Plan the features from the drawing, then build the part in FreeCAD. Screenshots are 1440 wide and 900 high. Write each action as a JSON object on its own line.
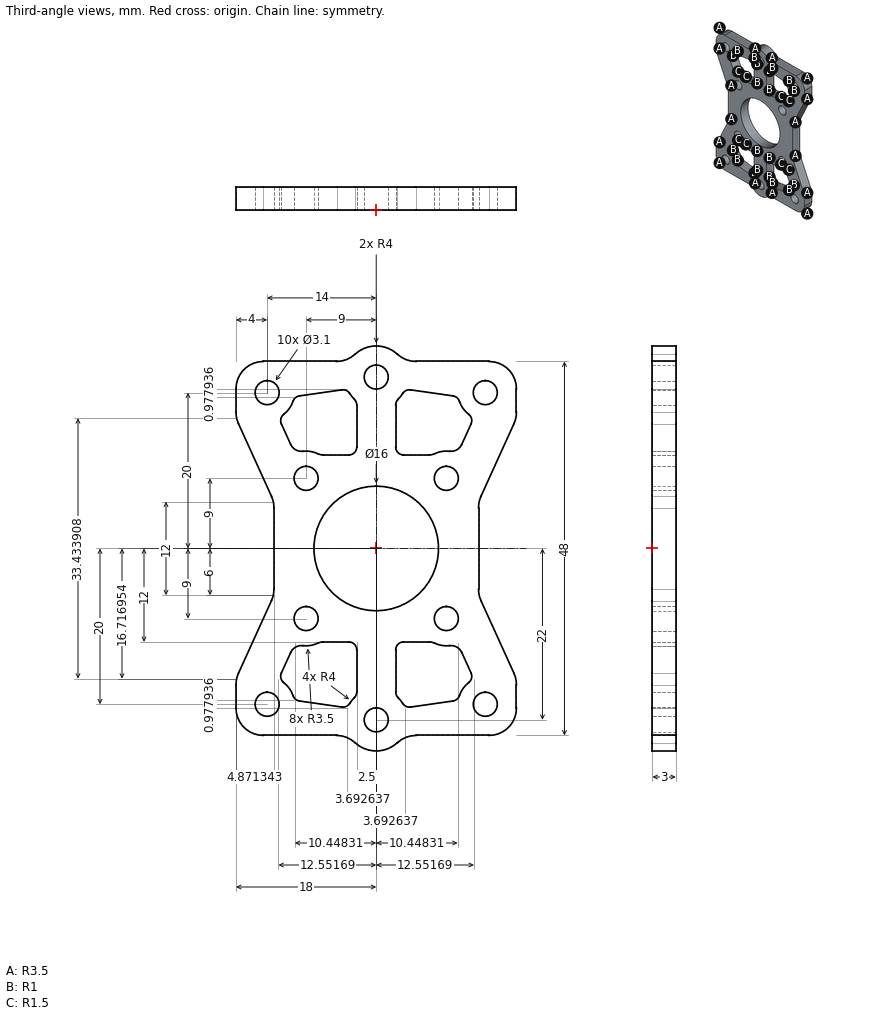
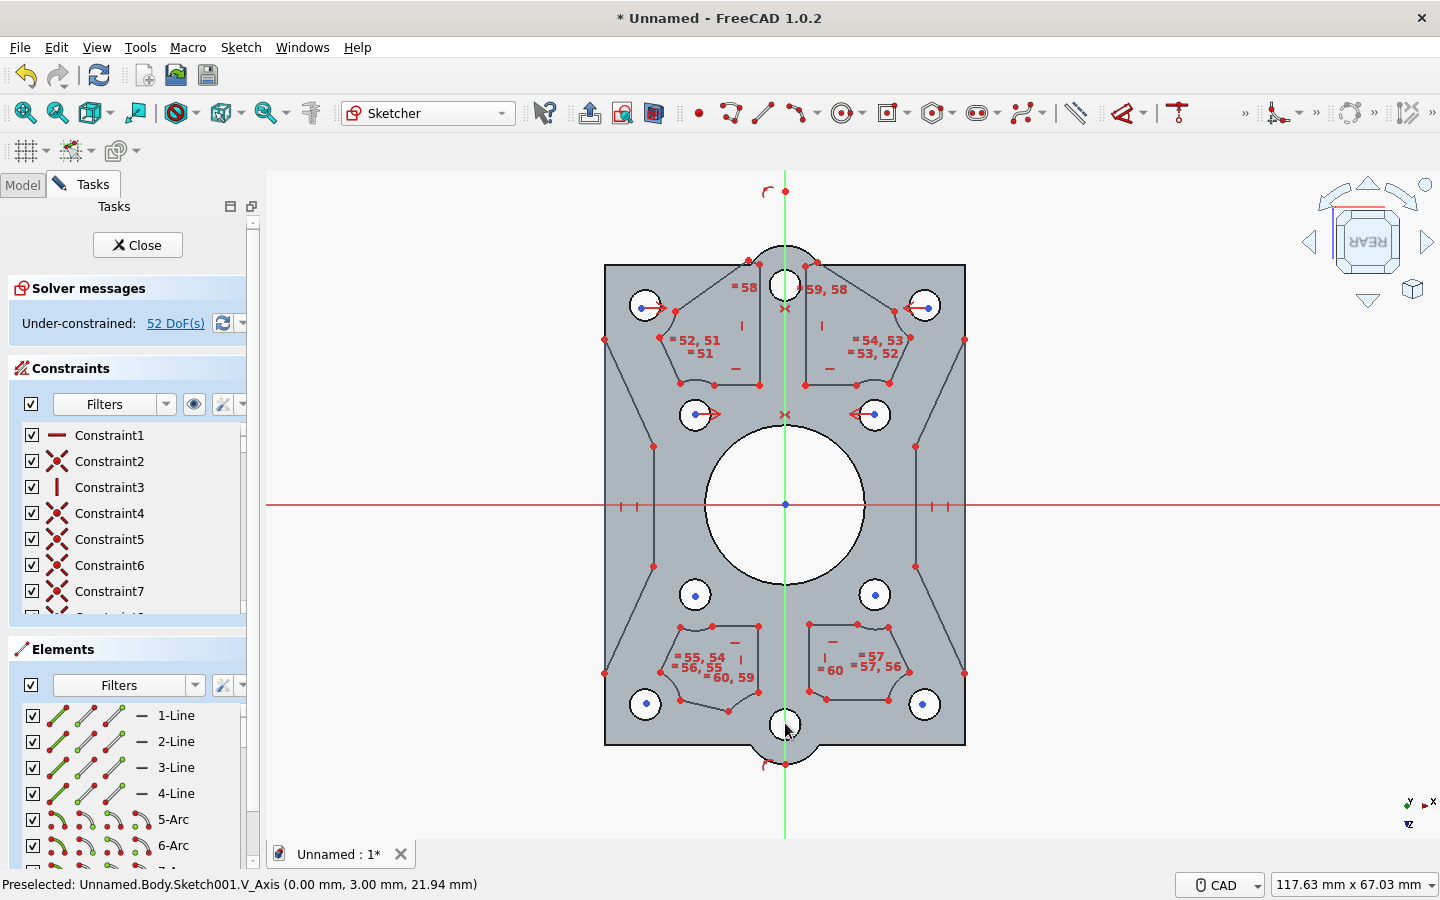
{"action": "left_click", "coordinate": [695, 414]}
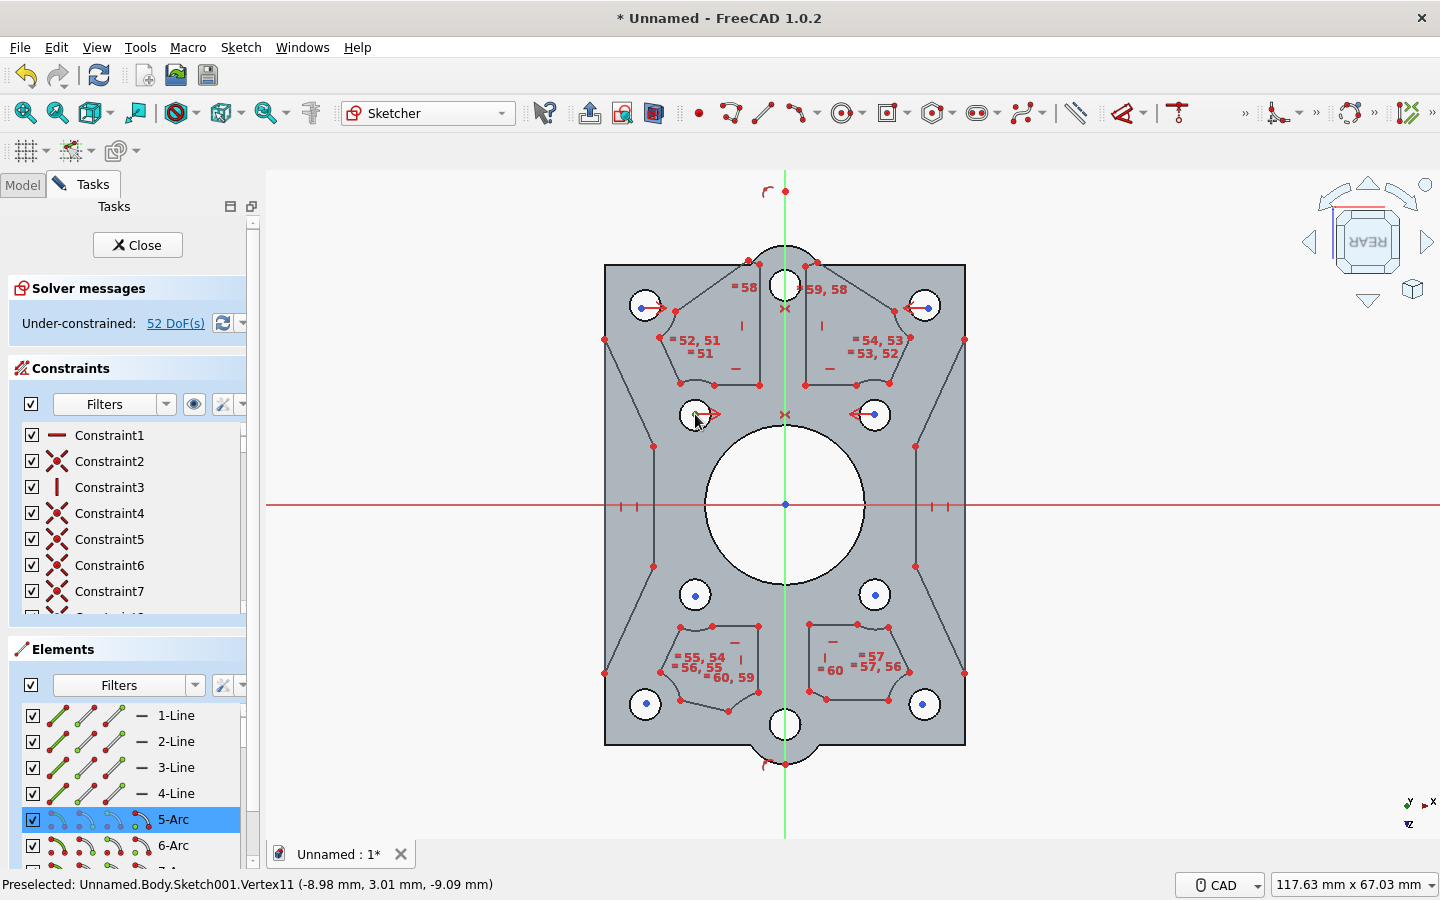
{"action": "left_click", "coordinate": [696, 596]}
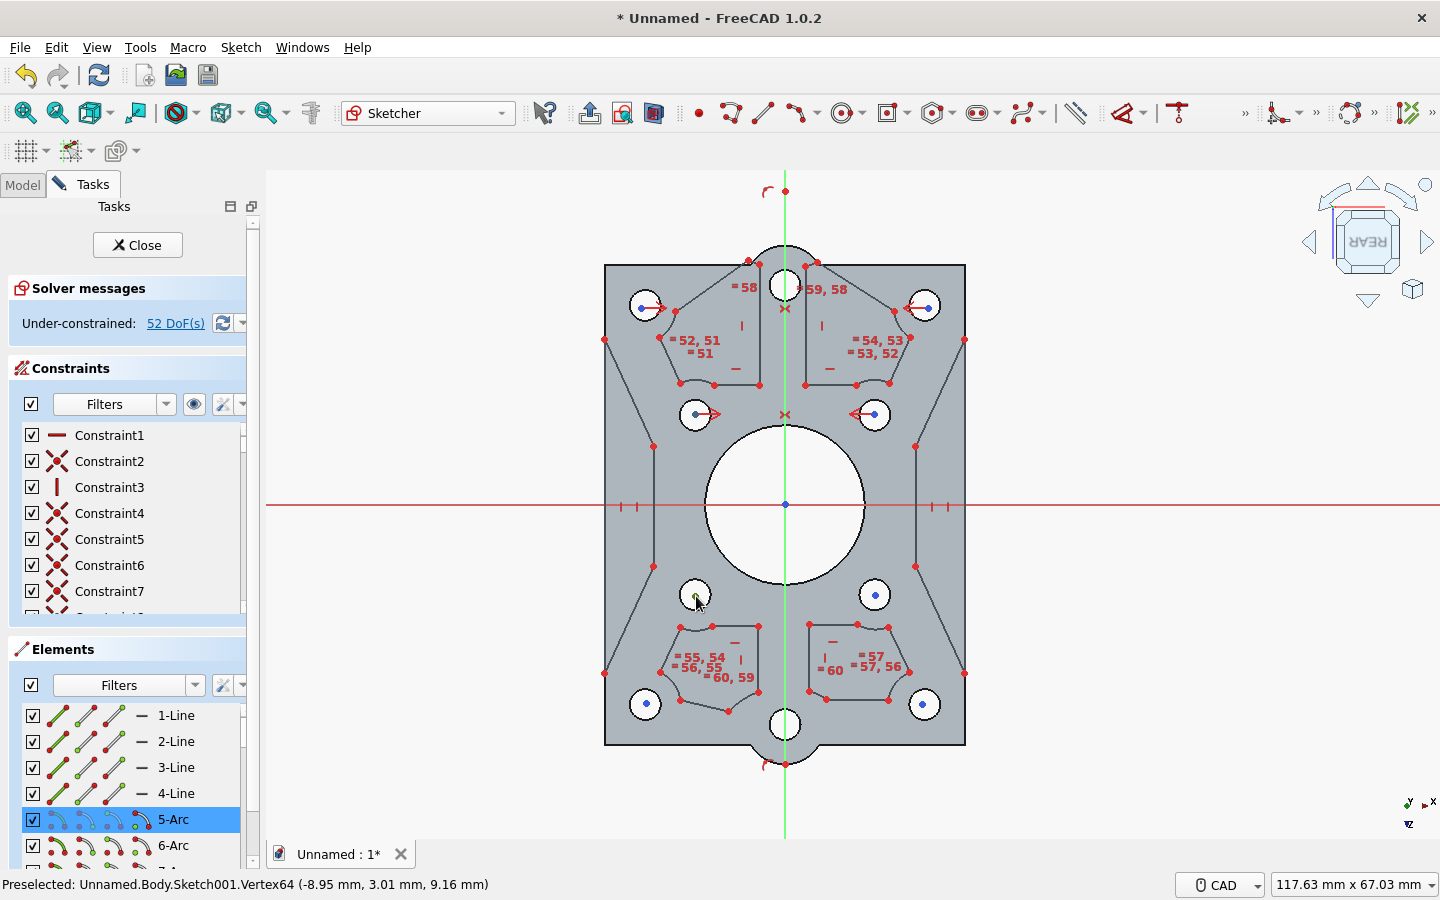
{"action": "left_click", "coordinate": [364, 505]}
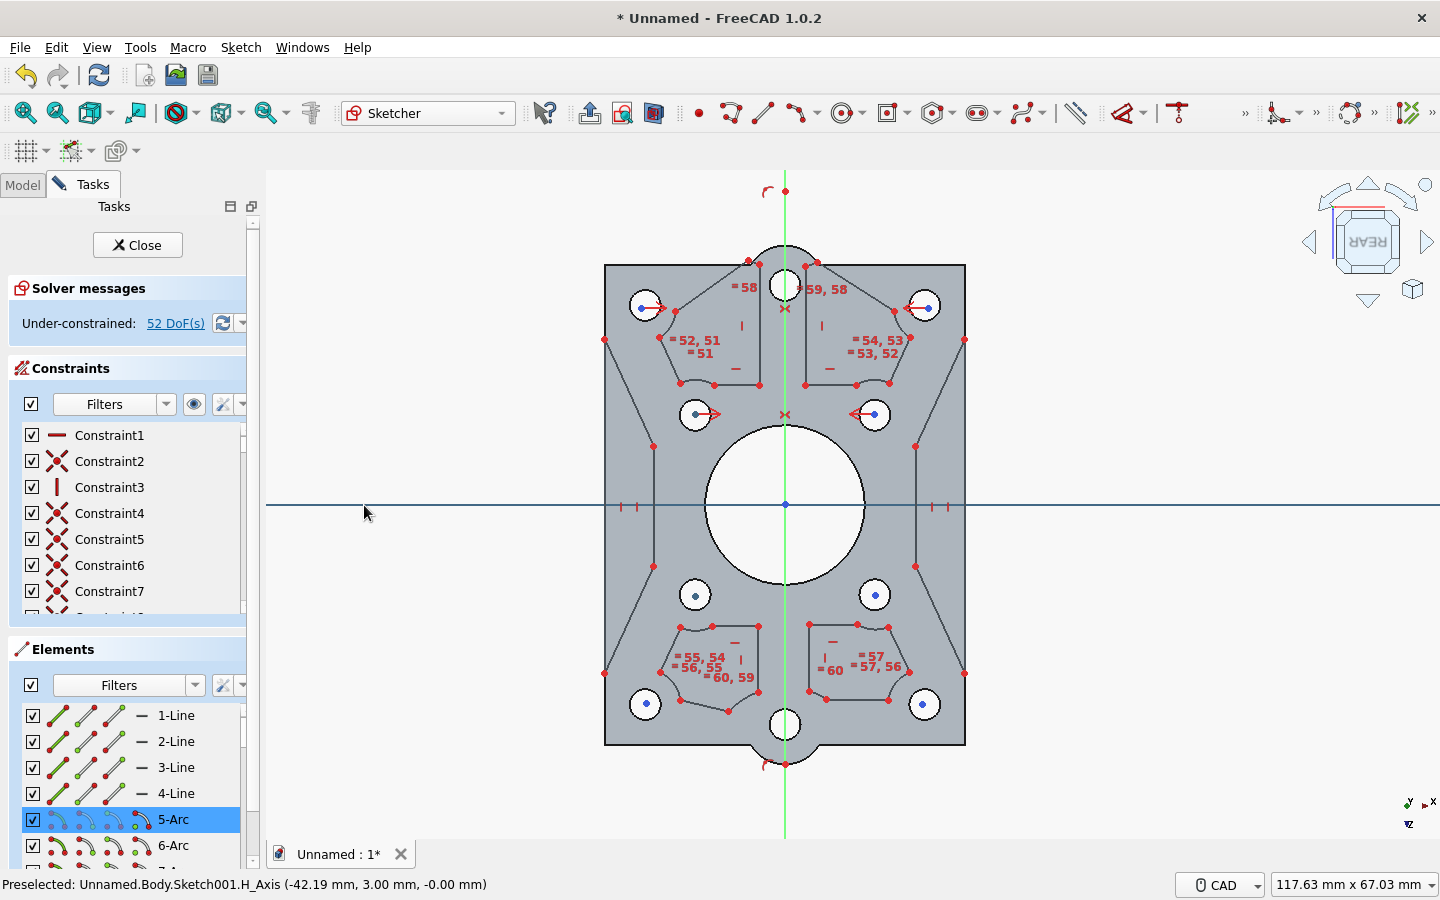
{"action": "key", "text": "s"}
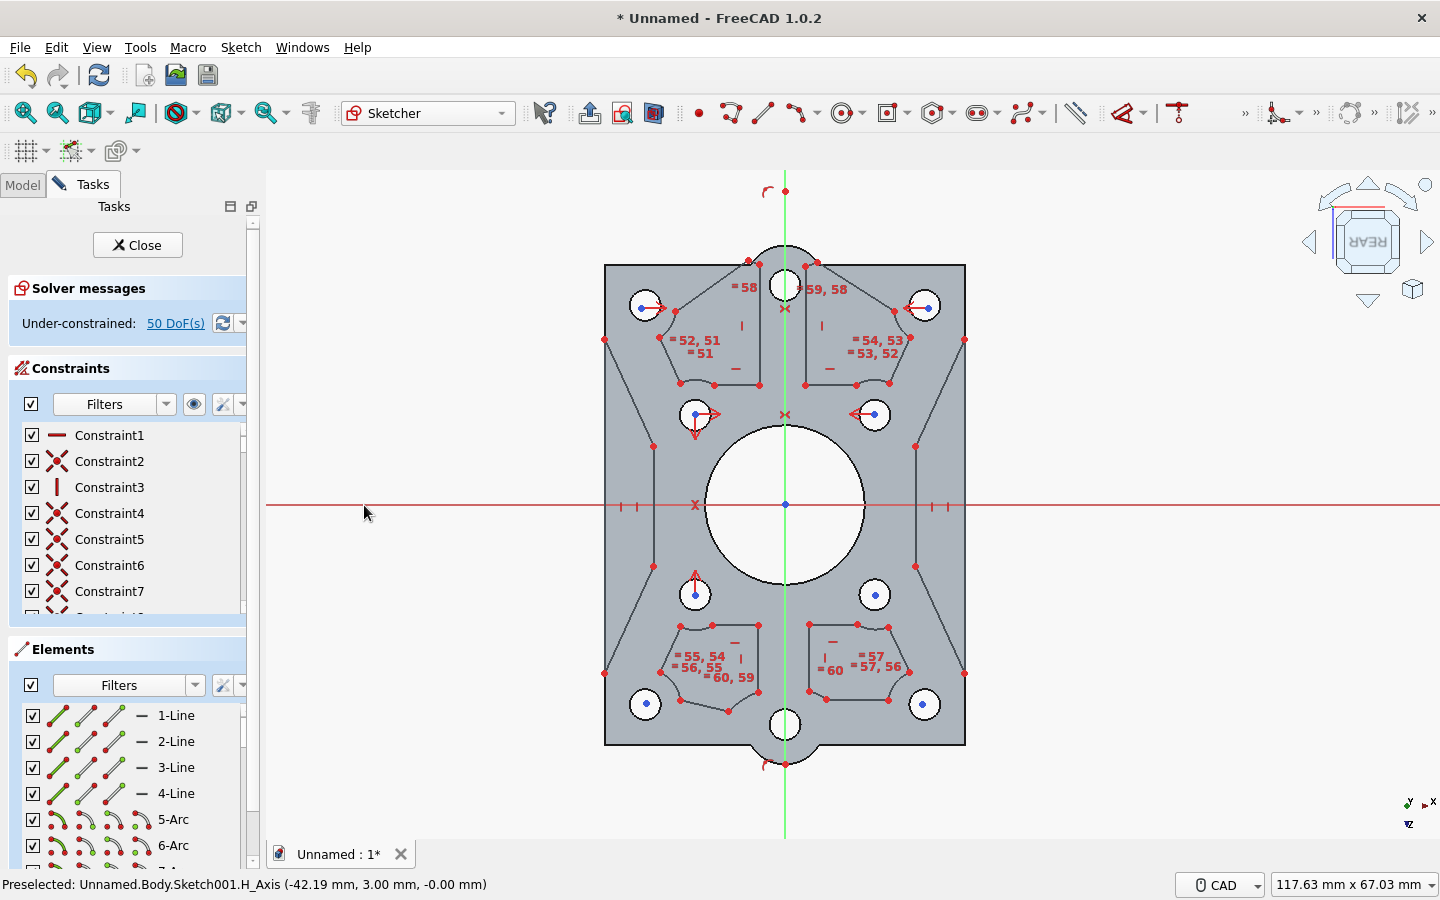
{"action": "left_click", "coordinate": [642, 308]}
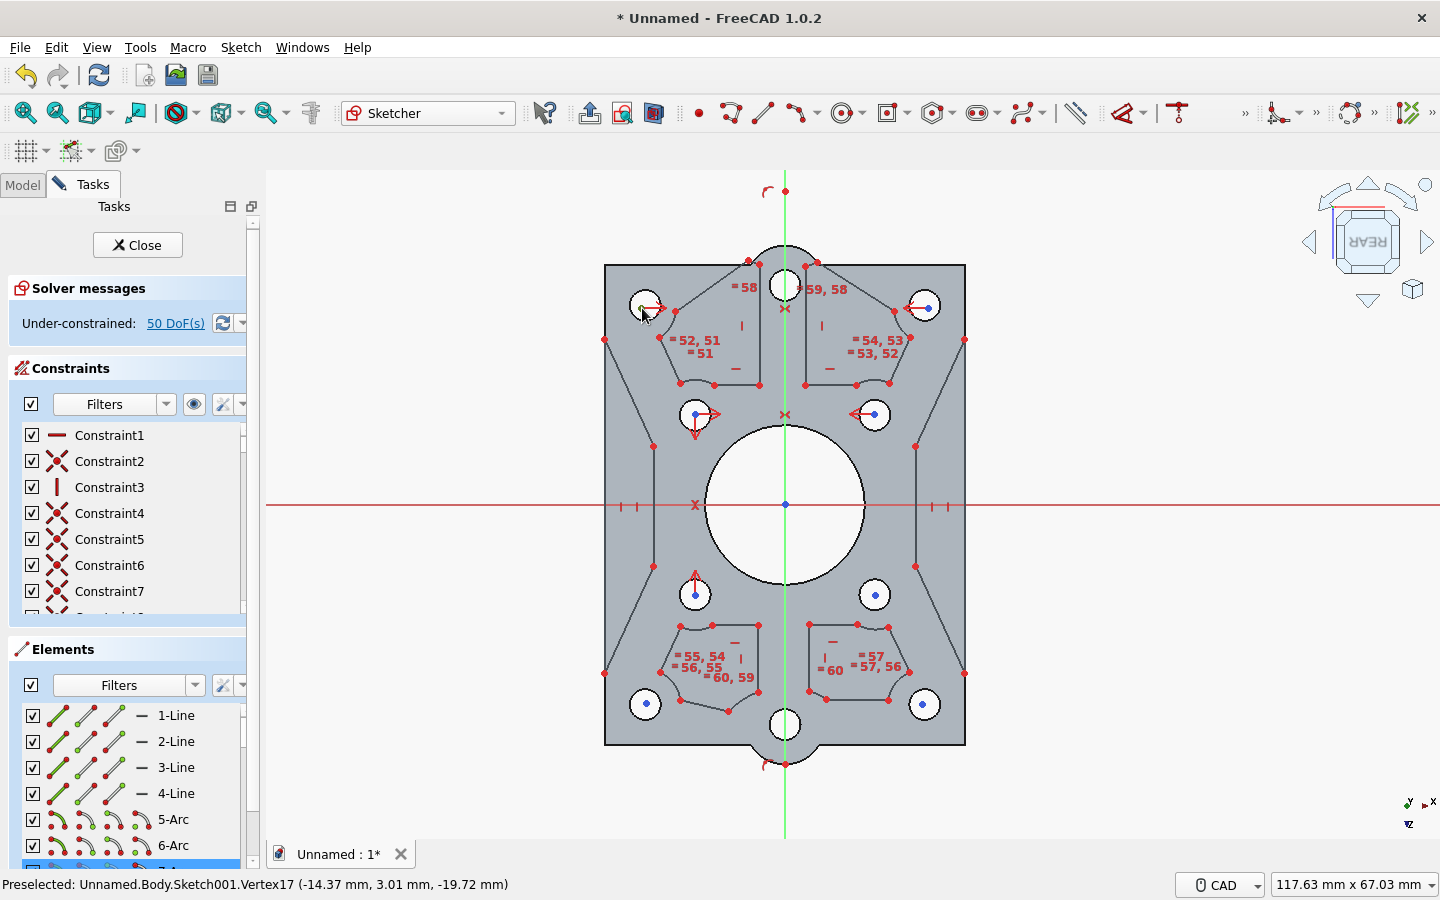
{"action": "left_click", "coordinate": [646, 704]}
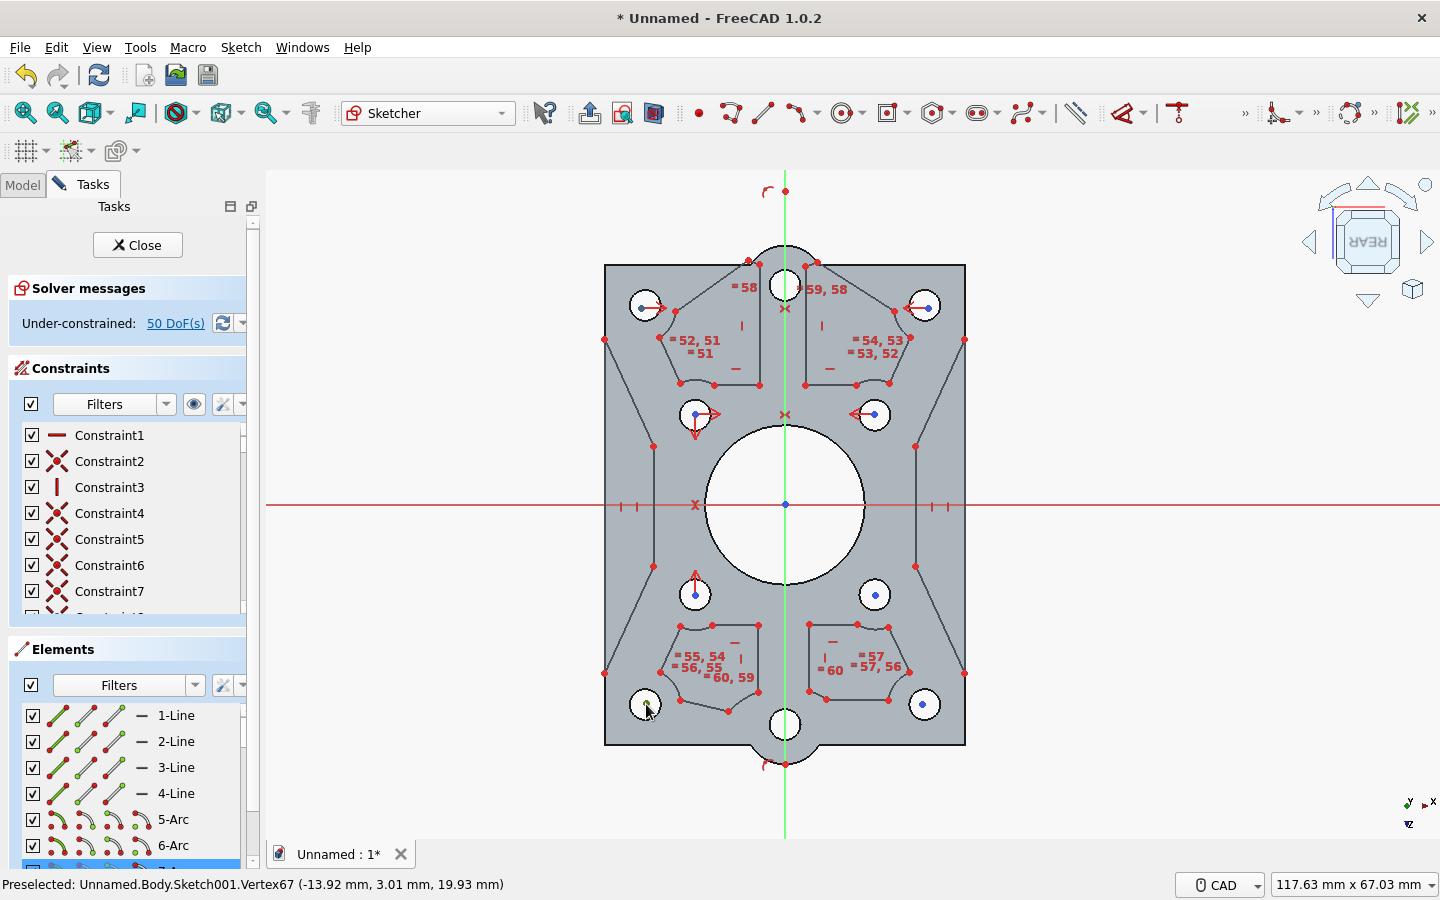
{"action": "left_click", "coordinate": [364, 505]}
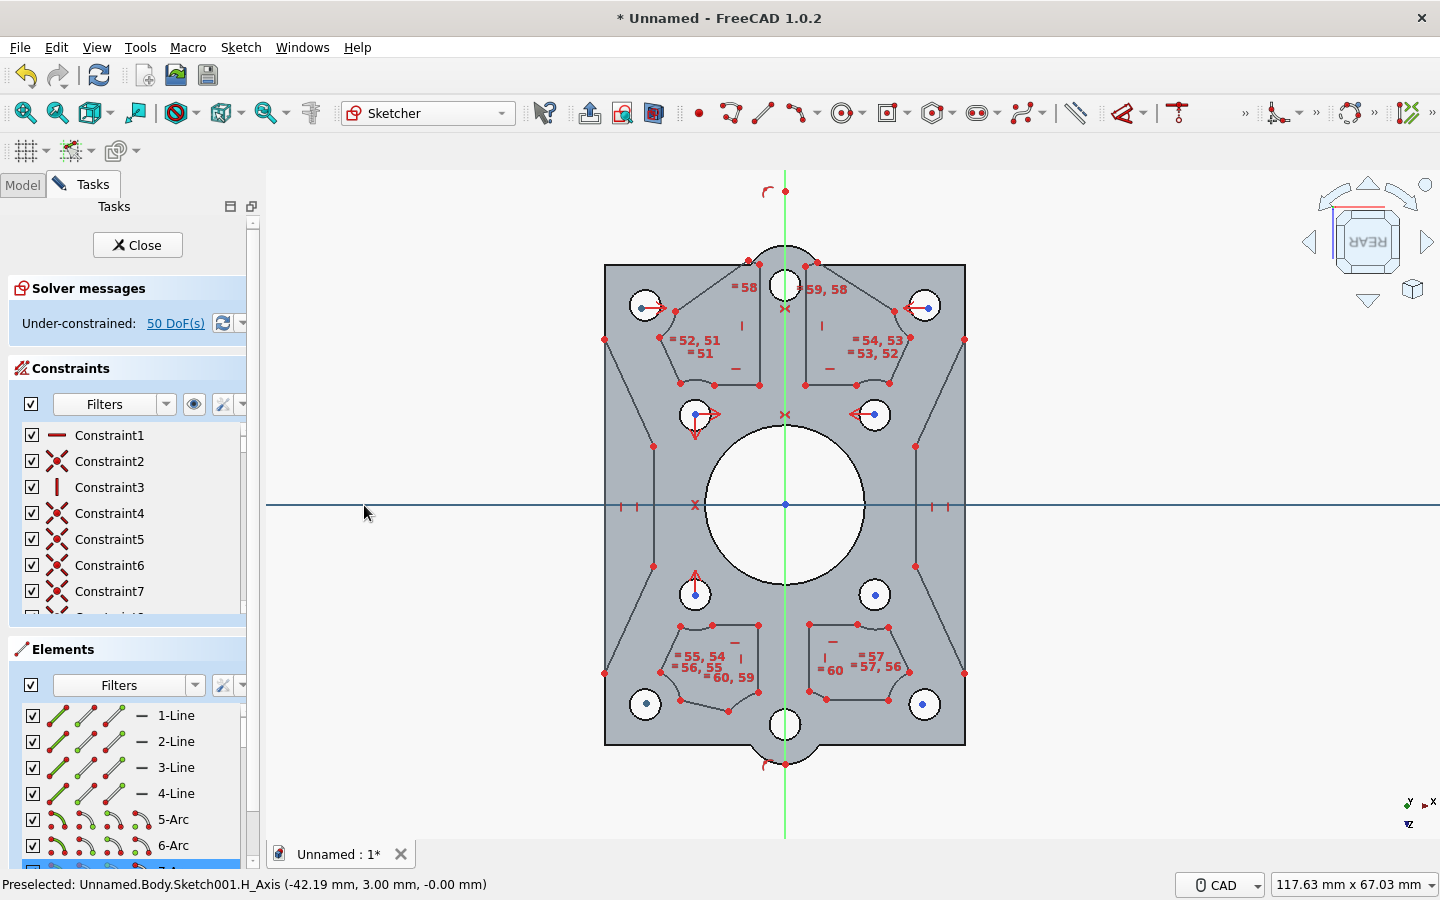
{"action": "key", "text": "s"}